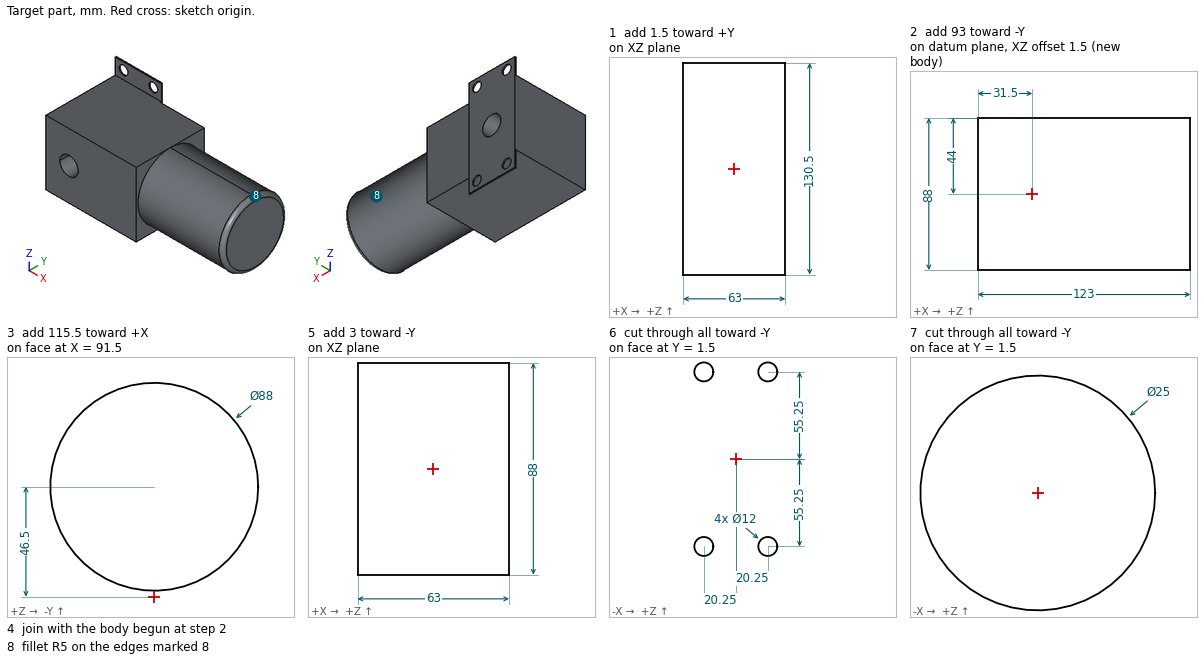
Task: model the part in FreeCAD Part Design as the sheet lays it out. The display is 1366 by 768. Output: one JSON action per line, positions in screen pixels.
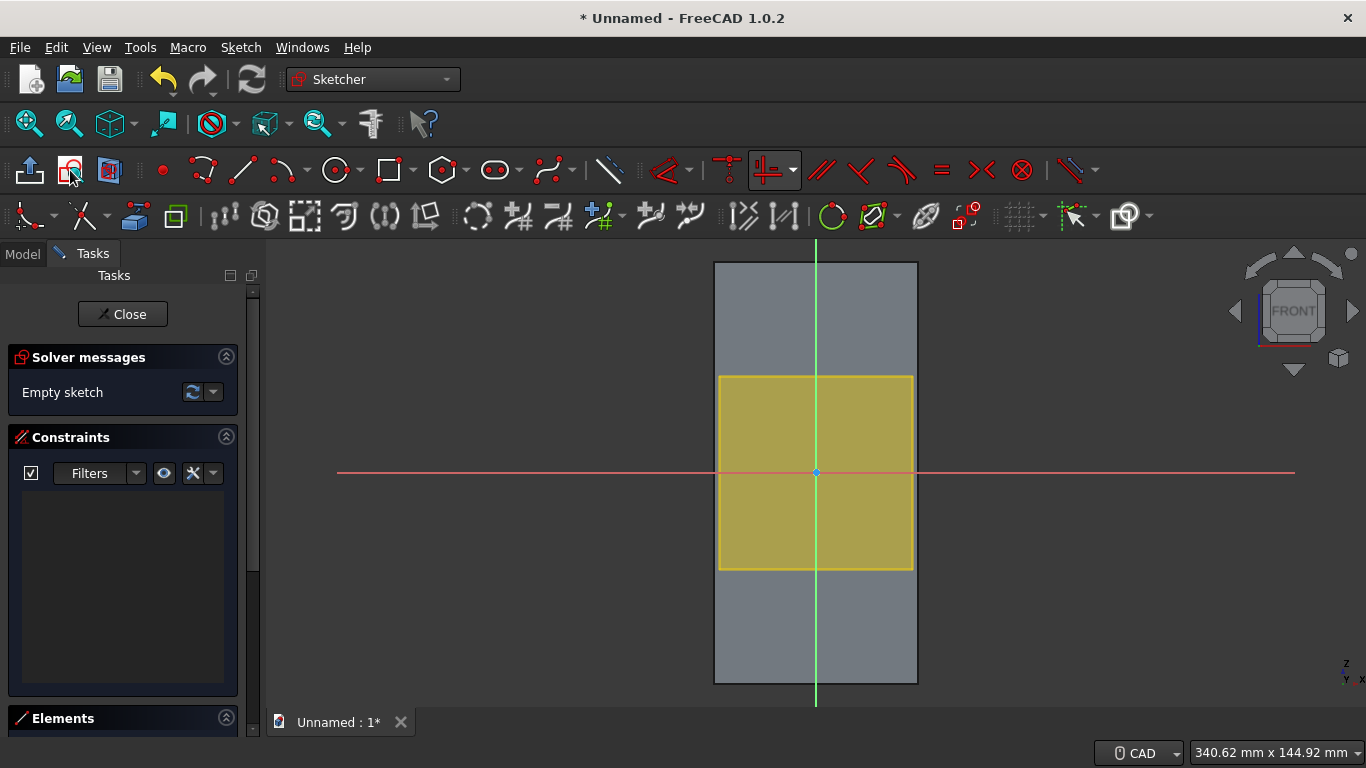
{"action": "left_click", "coordinate": [390, 170]}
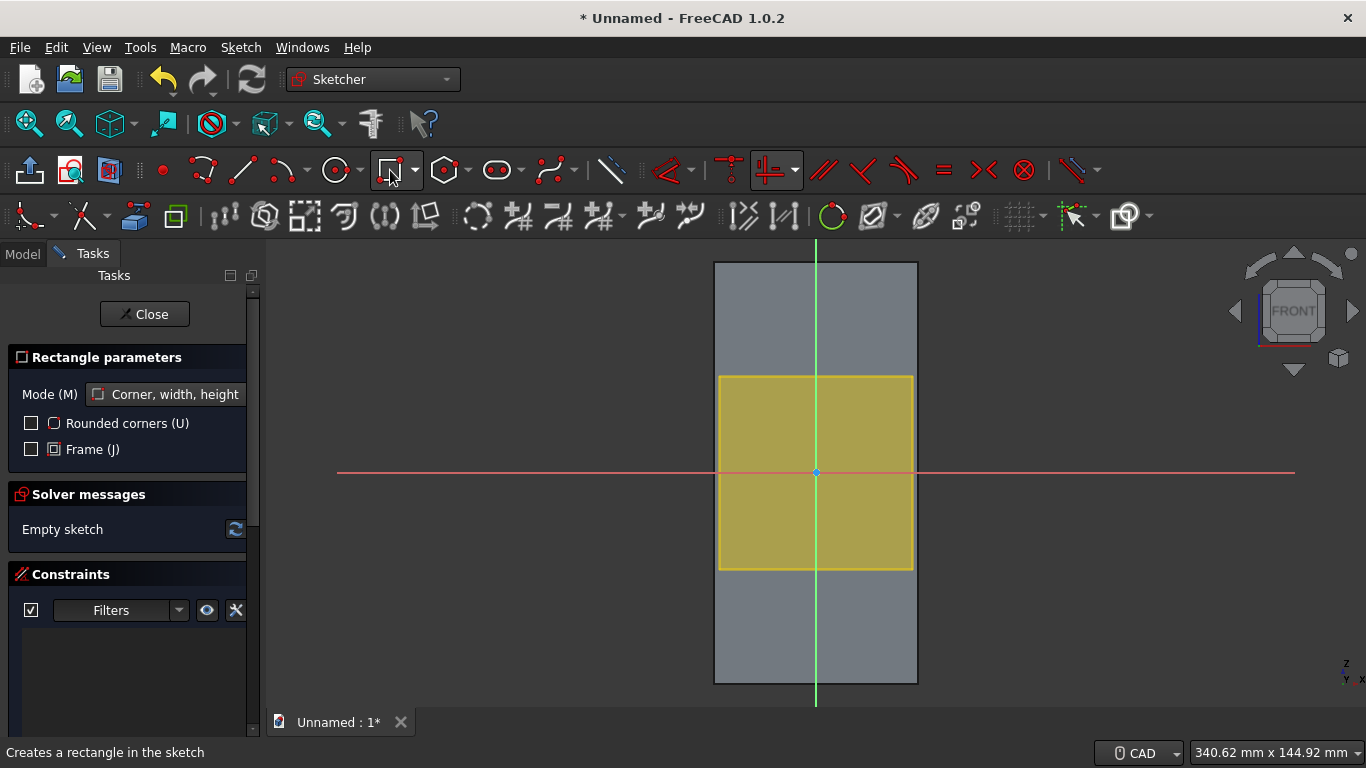
{"action": "left_click", "coordinate": [714, 331]}
{"action": "left_click", "coordinate": [1111, 615]}
{"action": "key", "text": "Escape"}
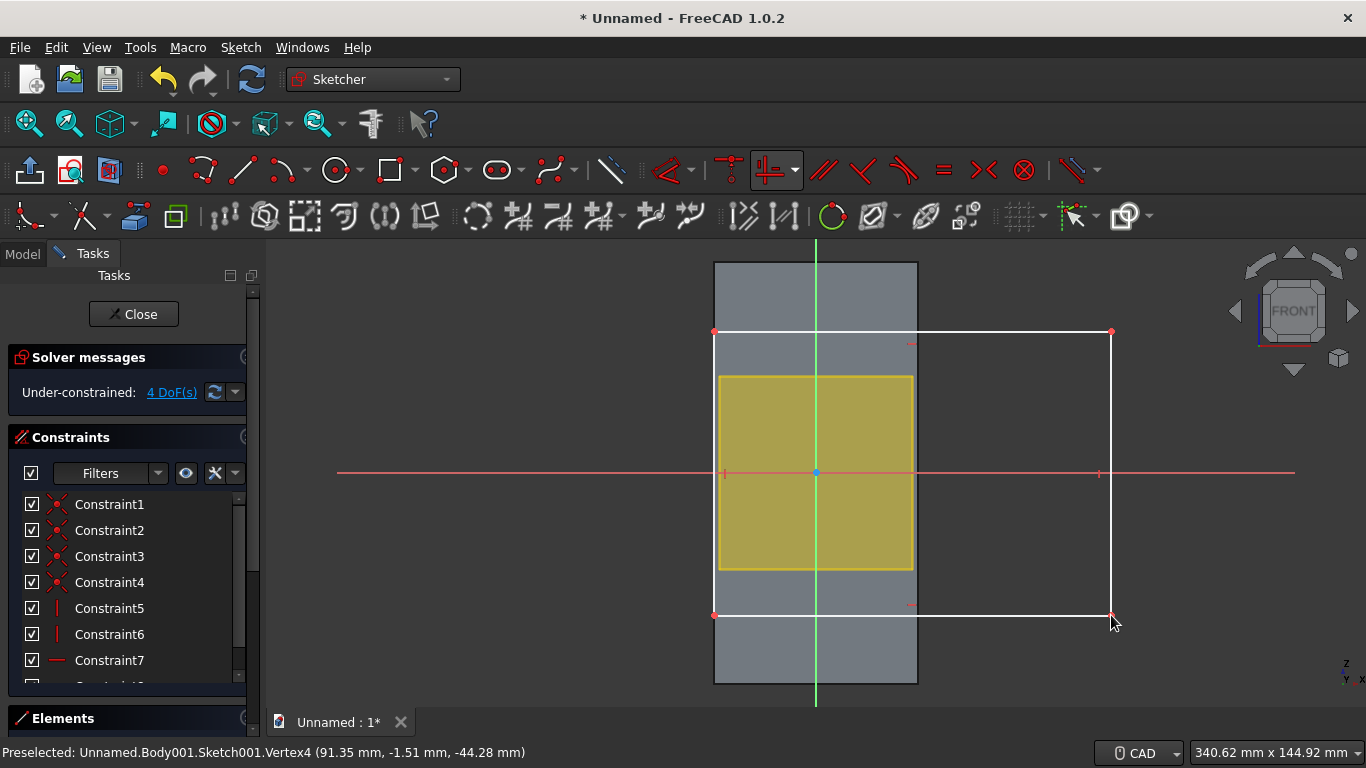
{"action": "left_click", "coordinate": [666, 170]}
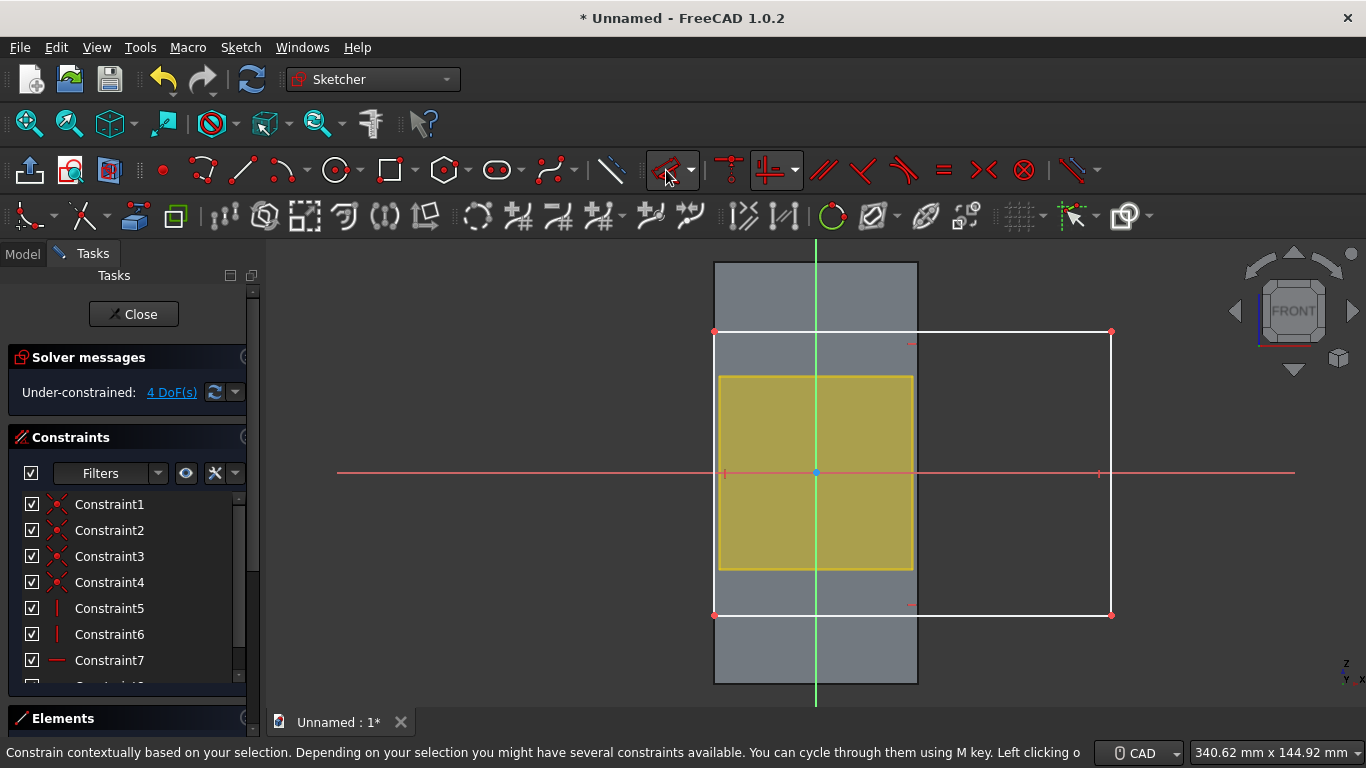
{"action": "left_click", "coordinate": [714, 417]}
{"action": "left_click", "coordinate": [680, 409]}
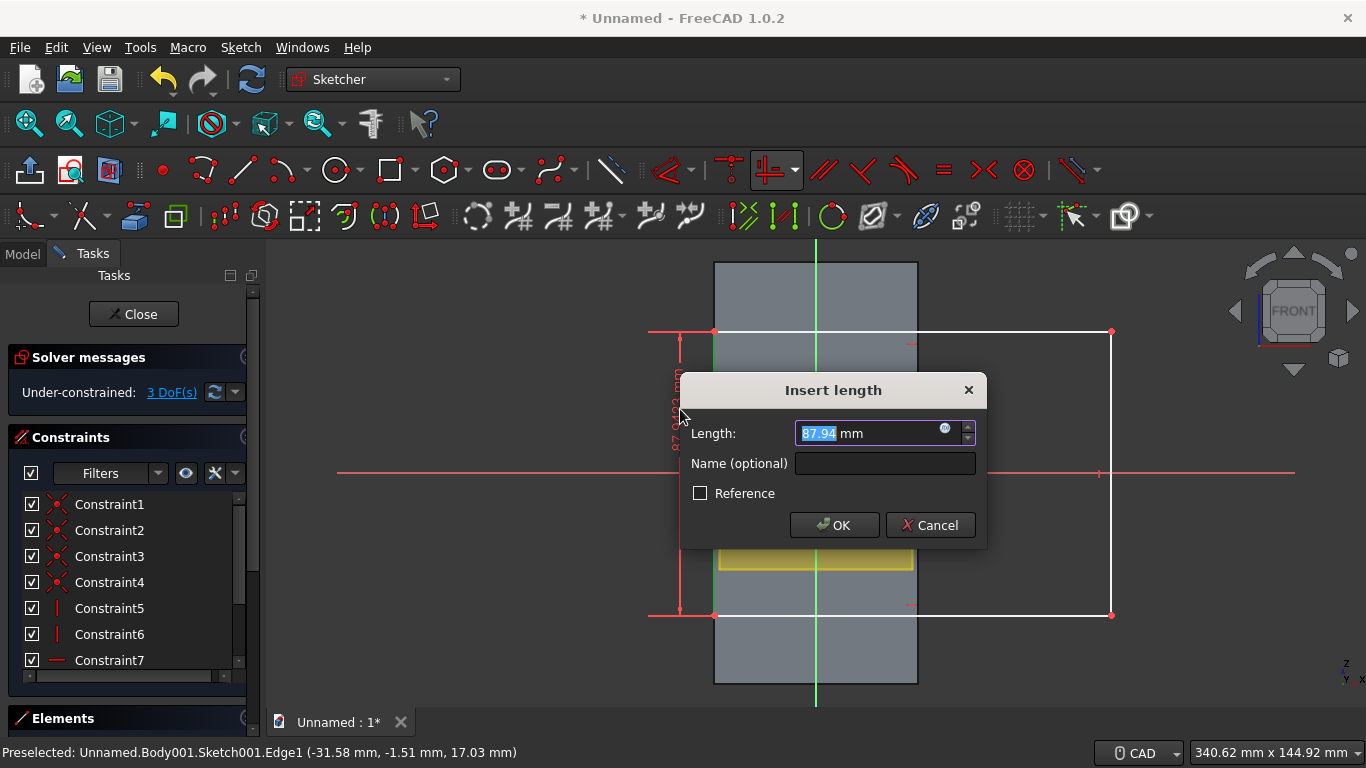
{"action": "type", "text": "88"}
{"action": "key", "text": "Return"}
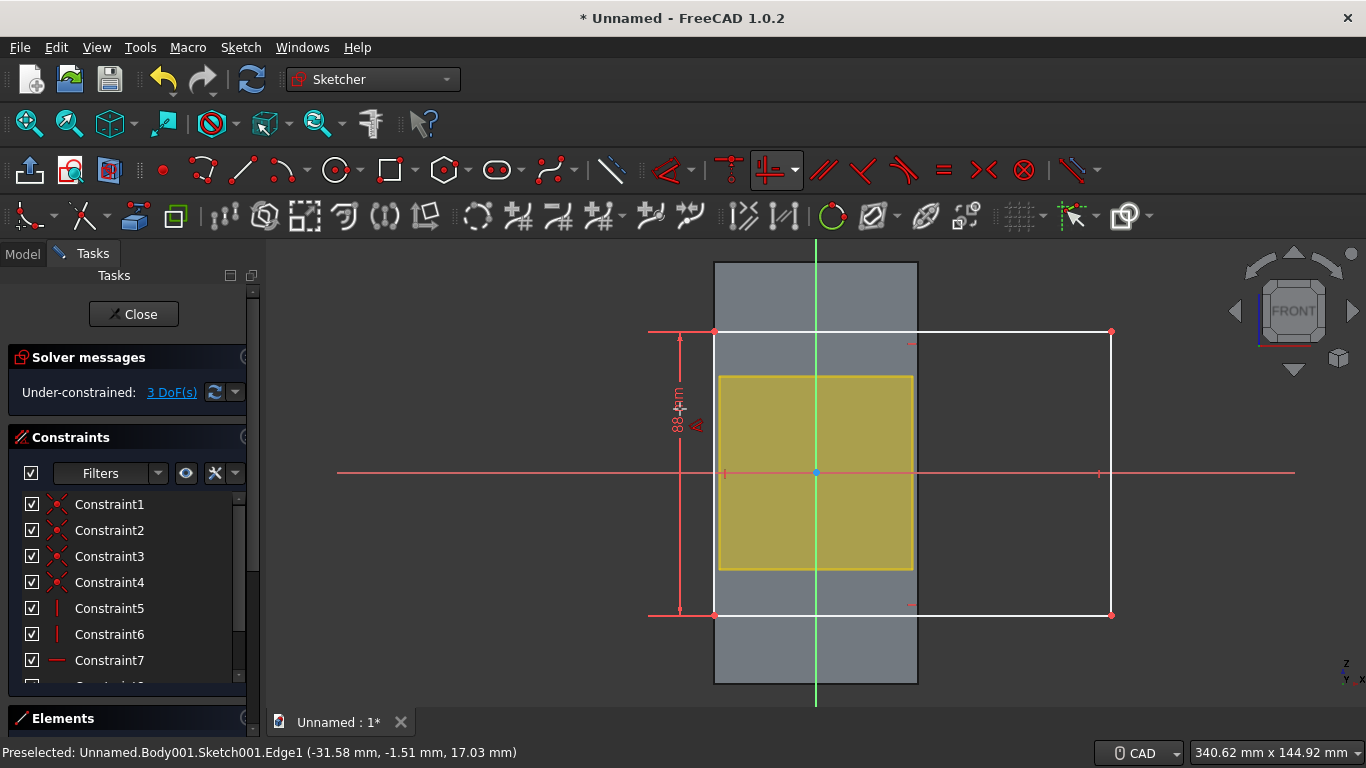
{"action": "left_click", "coordinate": [833, 616]}
{"action": "left_click", "coordinate": [912, 650]}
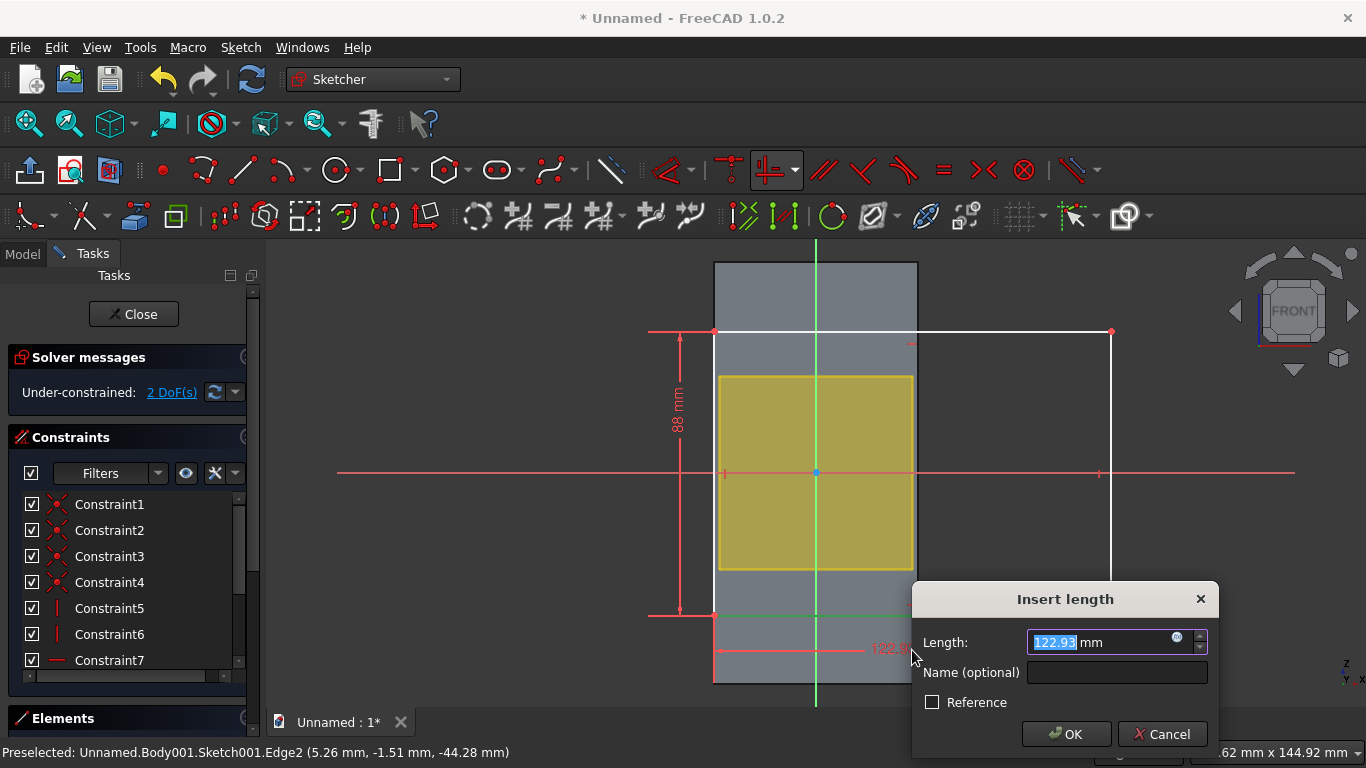
{"action": "type", "text": "123"}
{"action": "key", "text": "Return"}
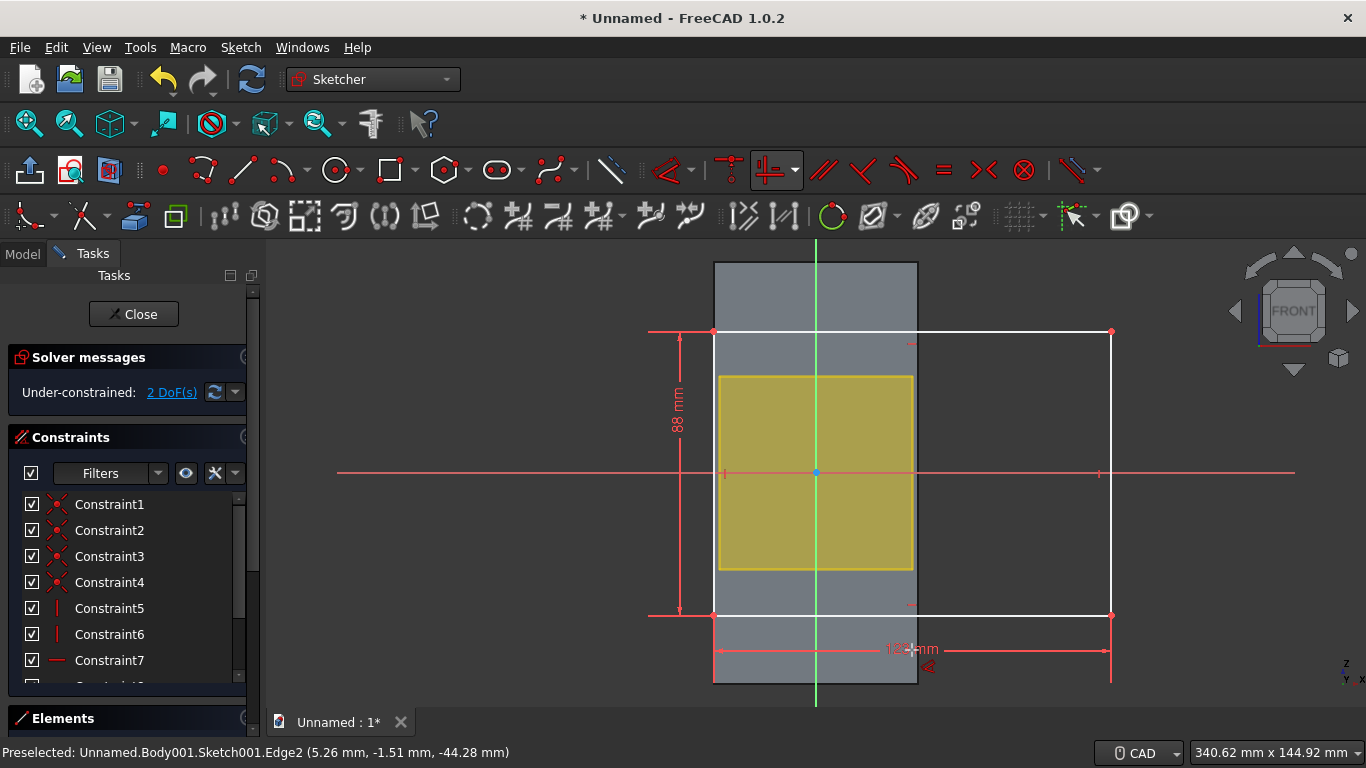
{"action": "left_click", "coordinate": [714, 332]}
{"action": "left_click", "coordinate": [680, 370]}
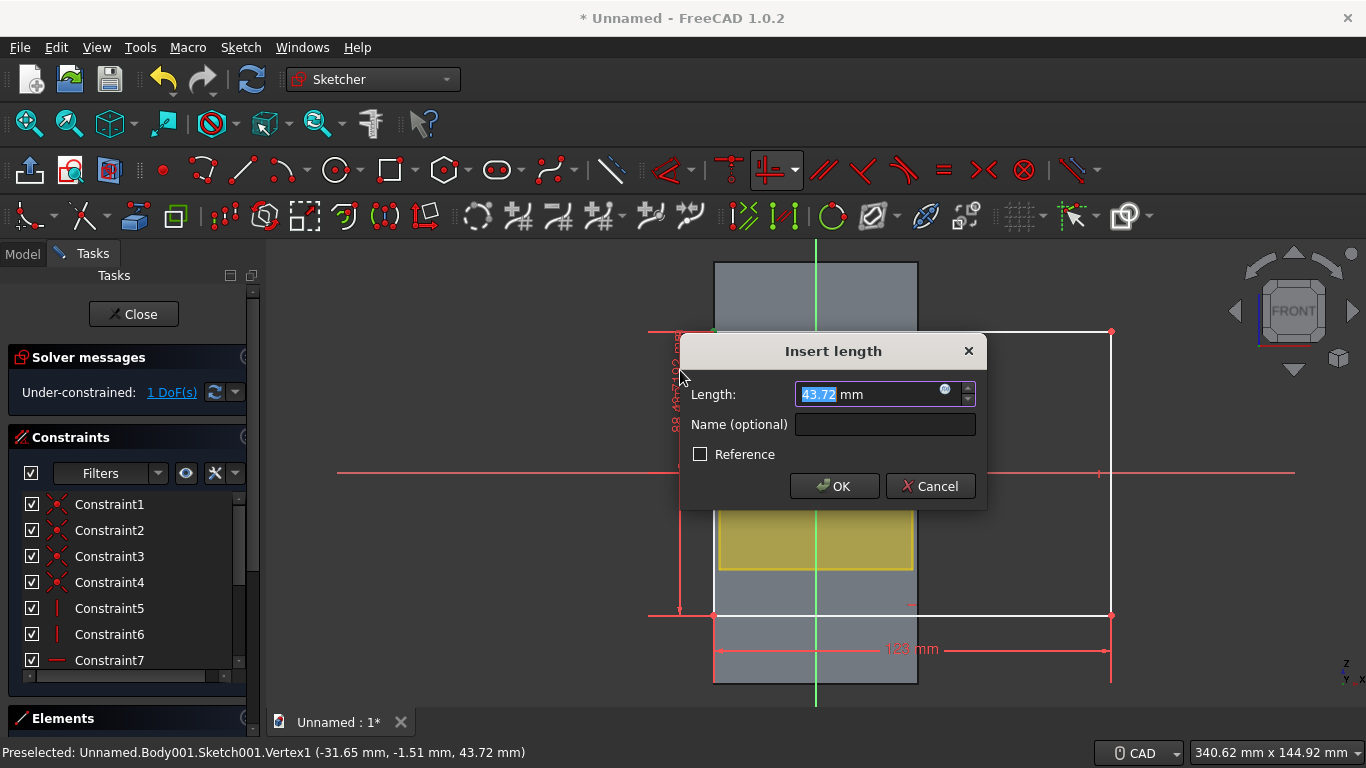
{"action": "type", "text": "44"}
{"action": "key", "text": "Return"}